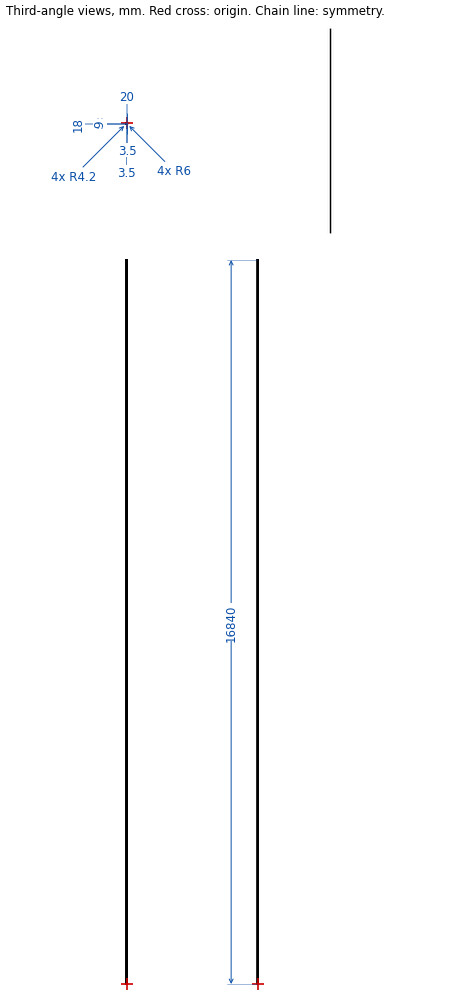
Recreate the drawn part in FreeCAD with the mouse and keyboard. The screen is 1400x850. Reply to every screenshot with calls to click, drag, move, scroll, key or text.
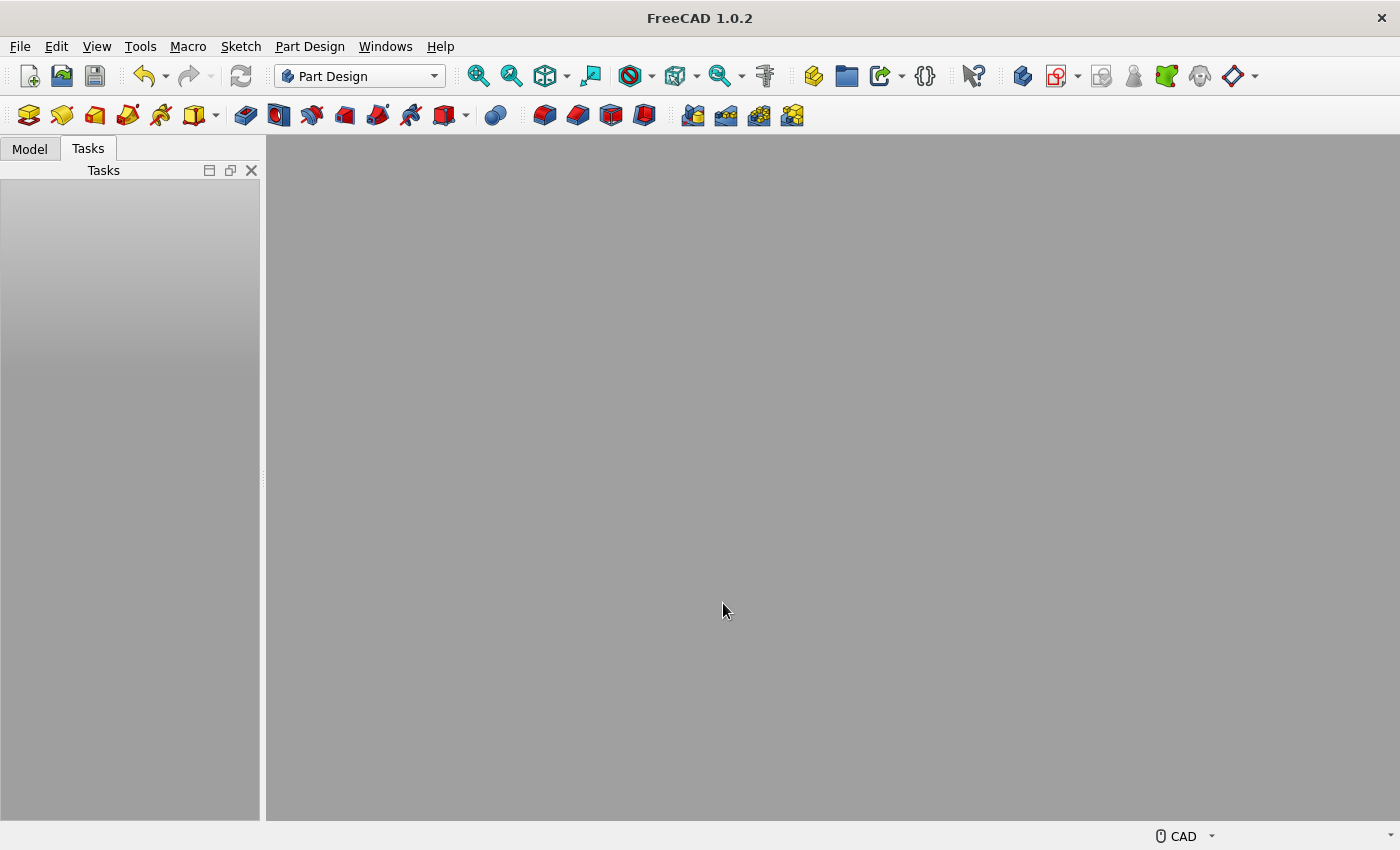
click(29, 76)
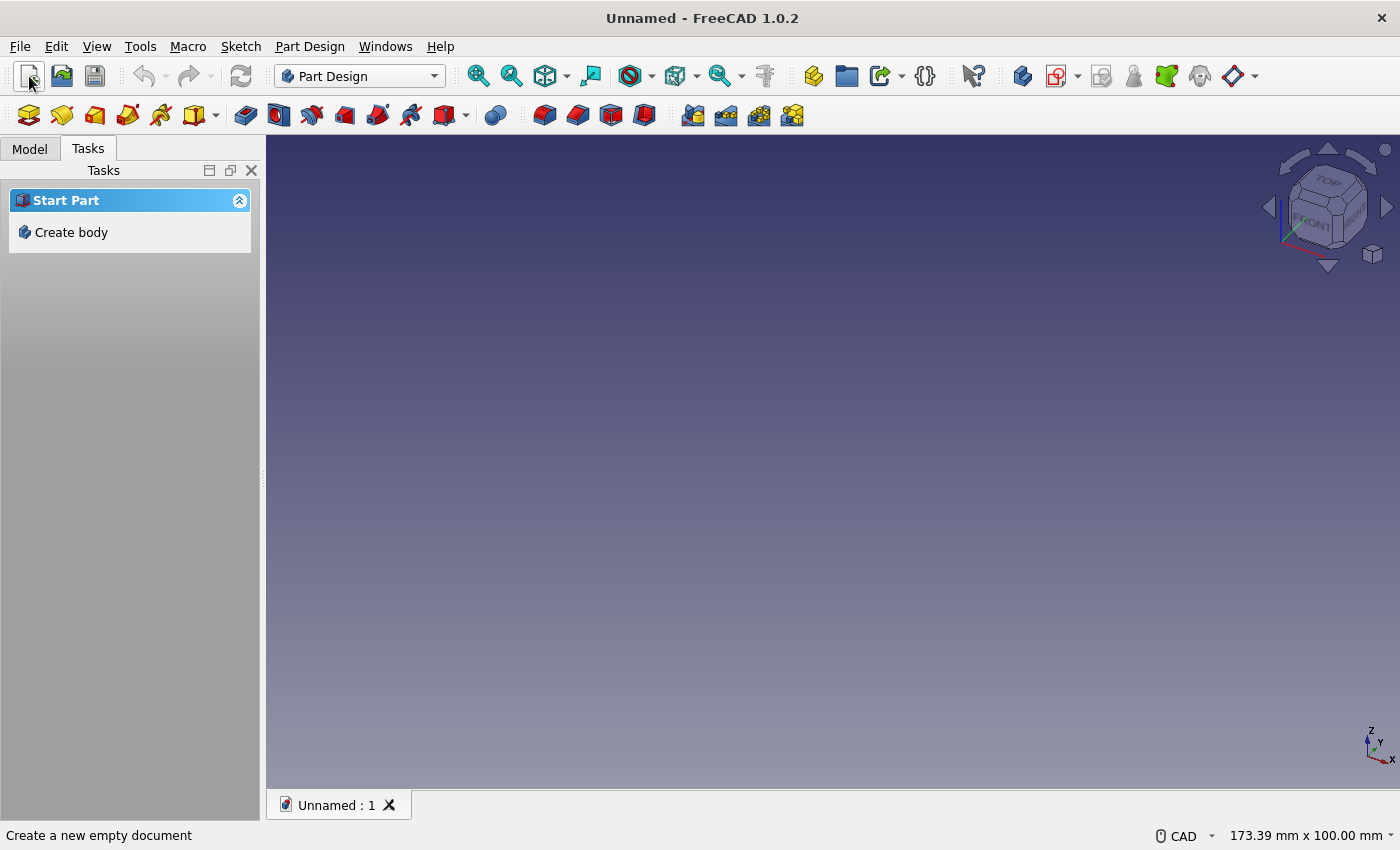
click(1056, 76)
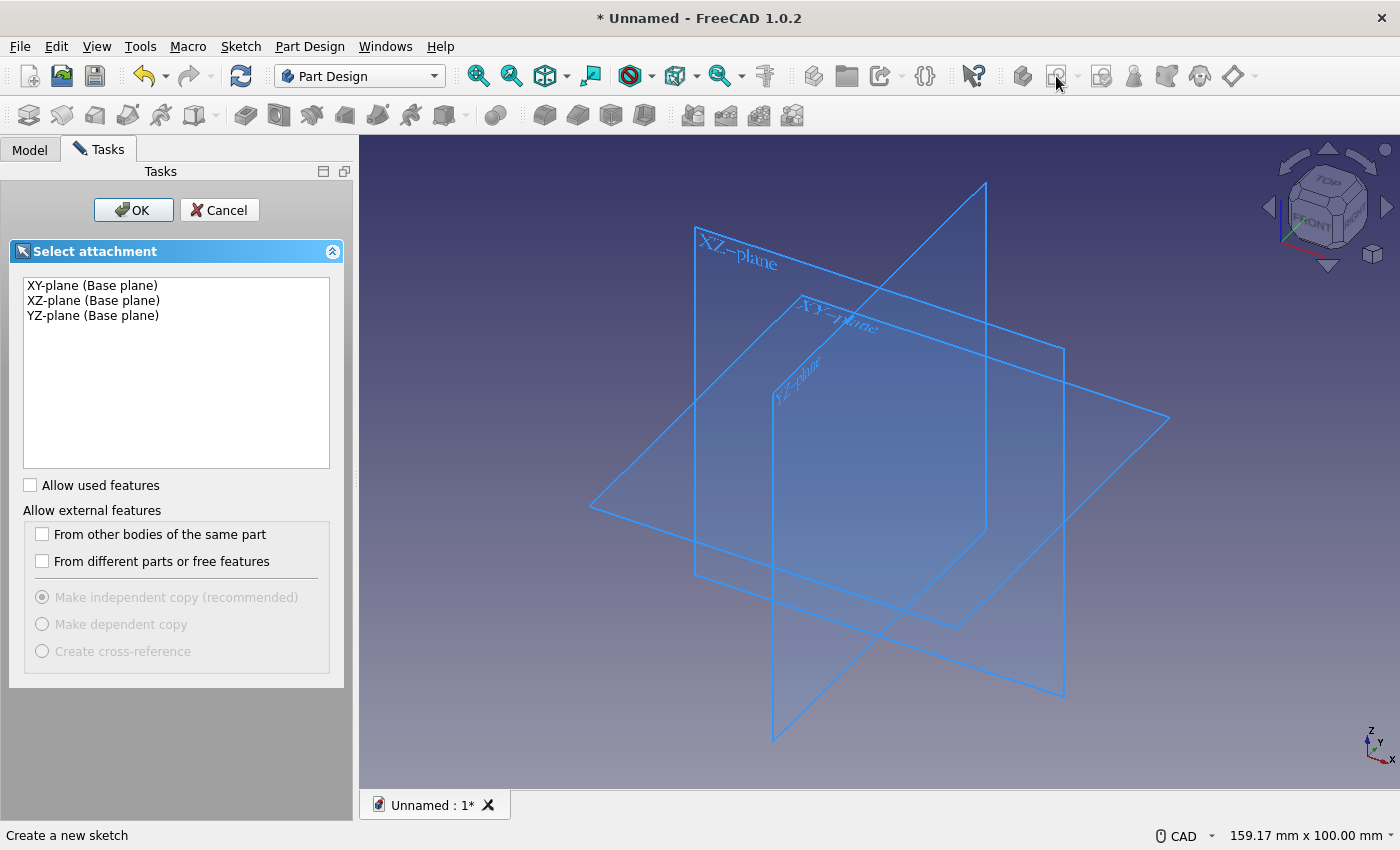
click(84, 286)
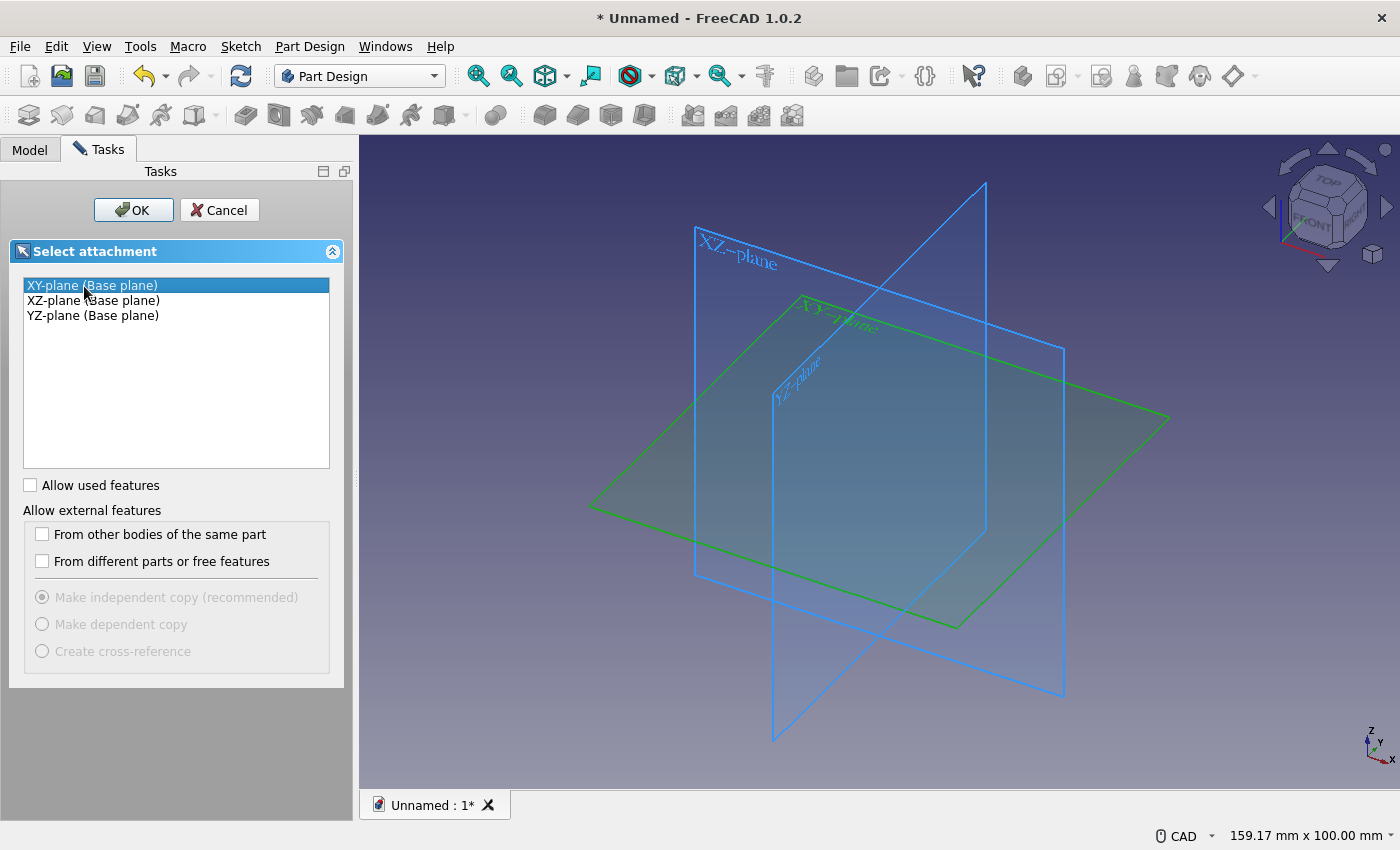
click(134, 210)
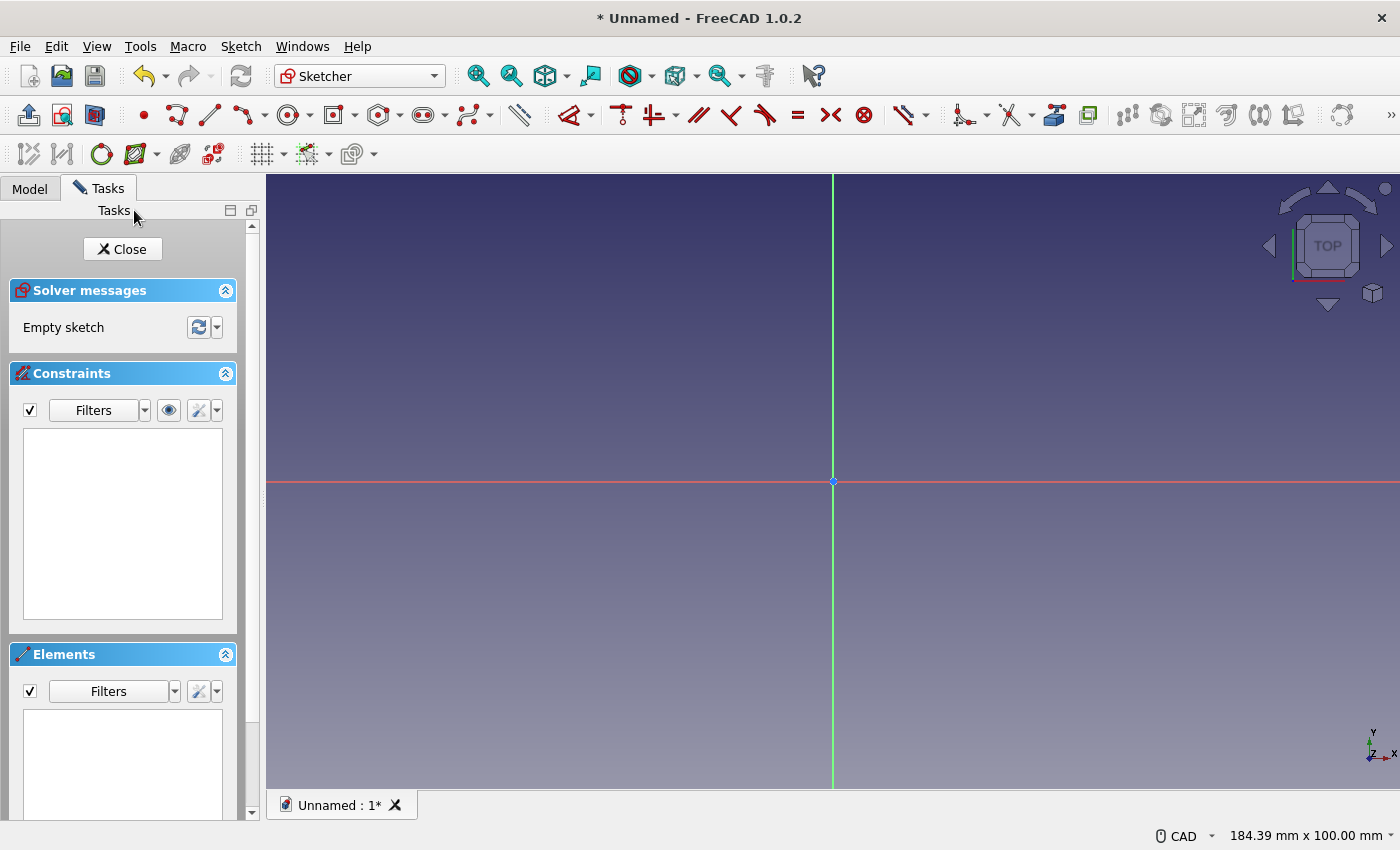
scroll(889, 482, up, 4)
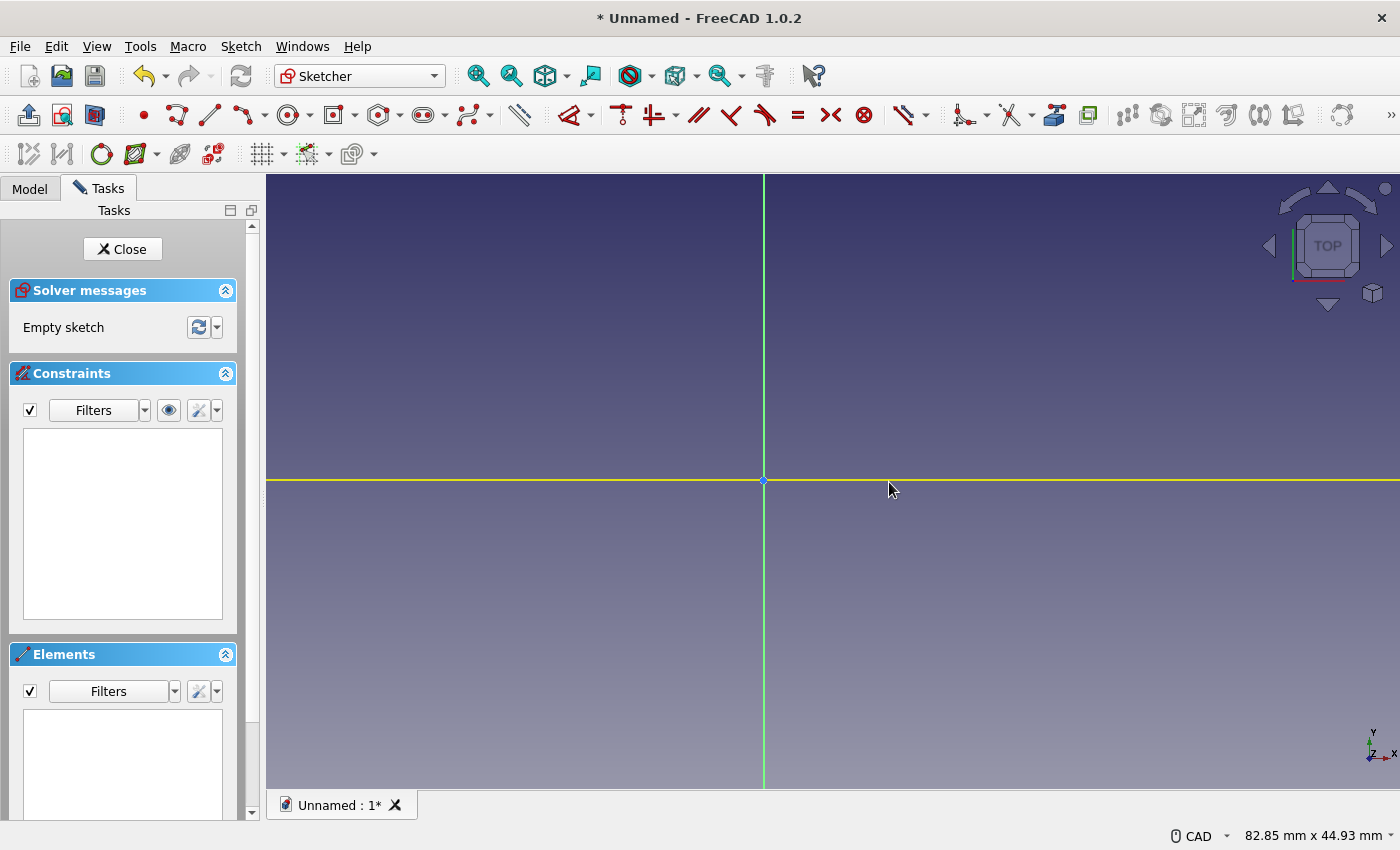
click(210, 116)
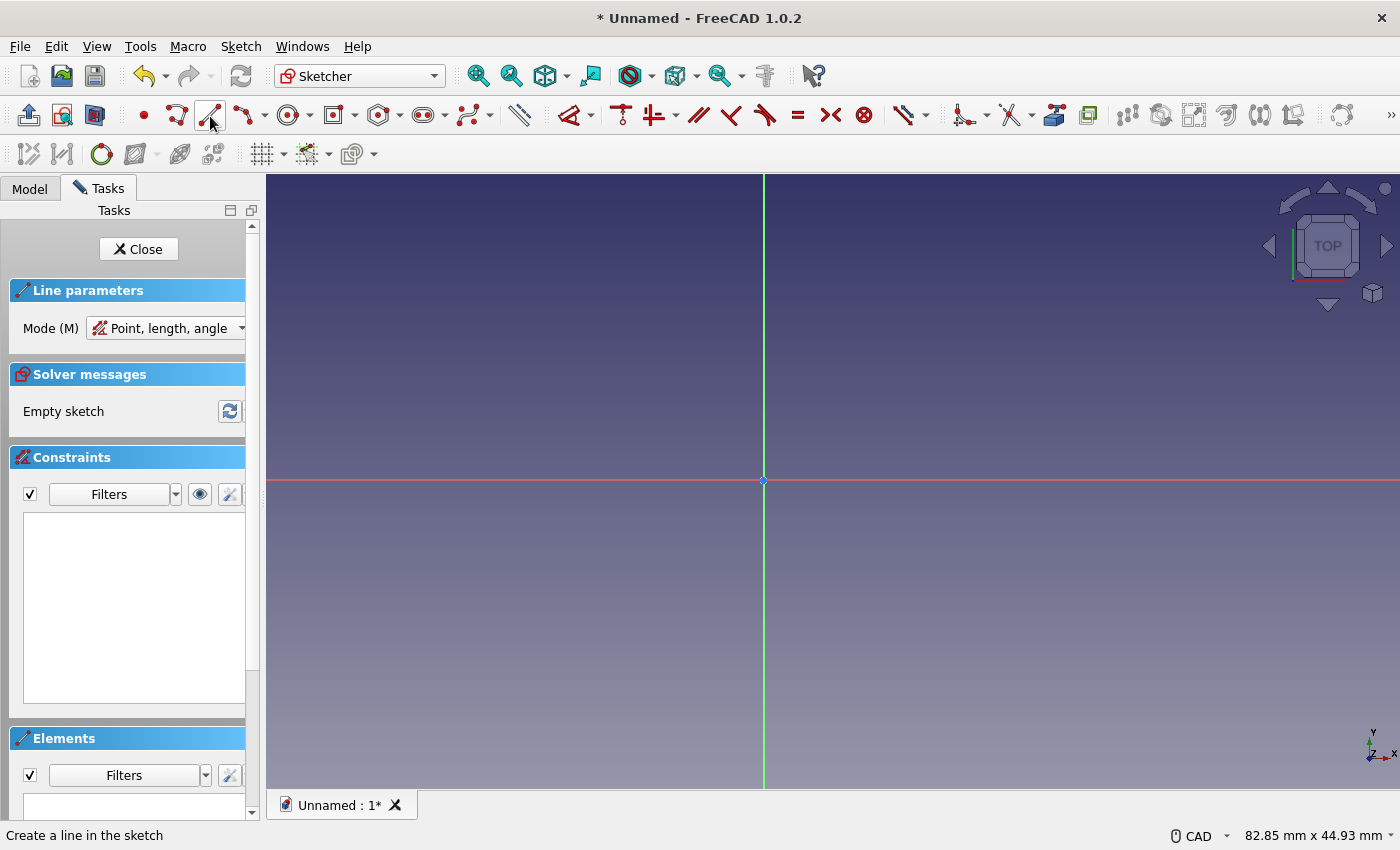
click(569, 603)
click(569, 357)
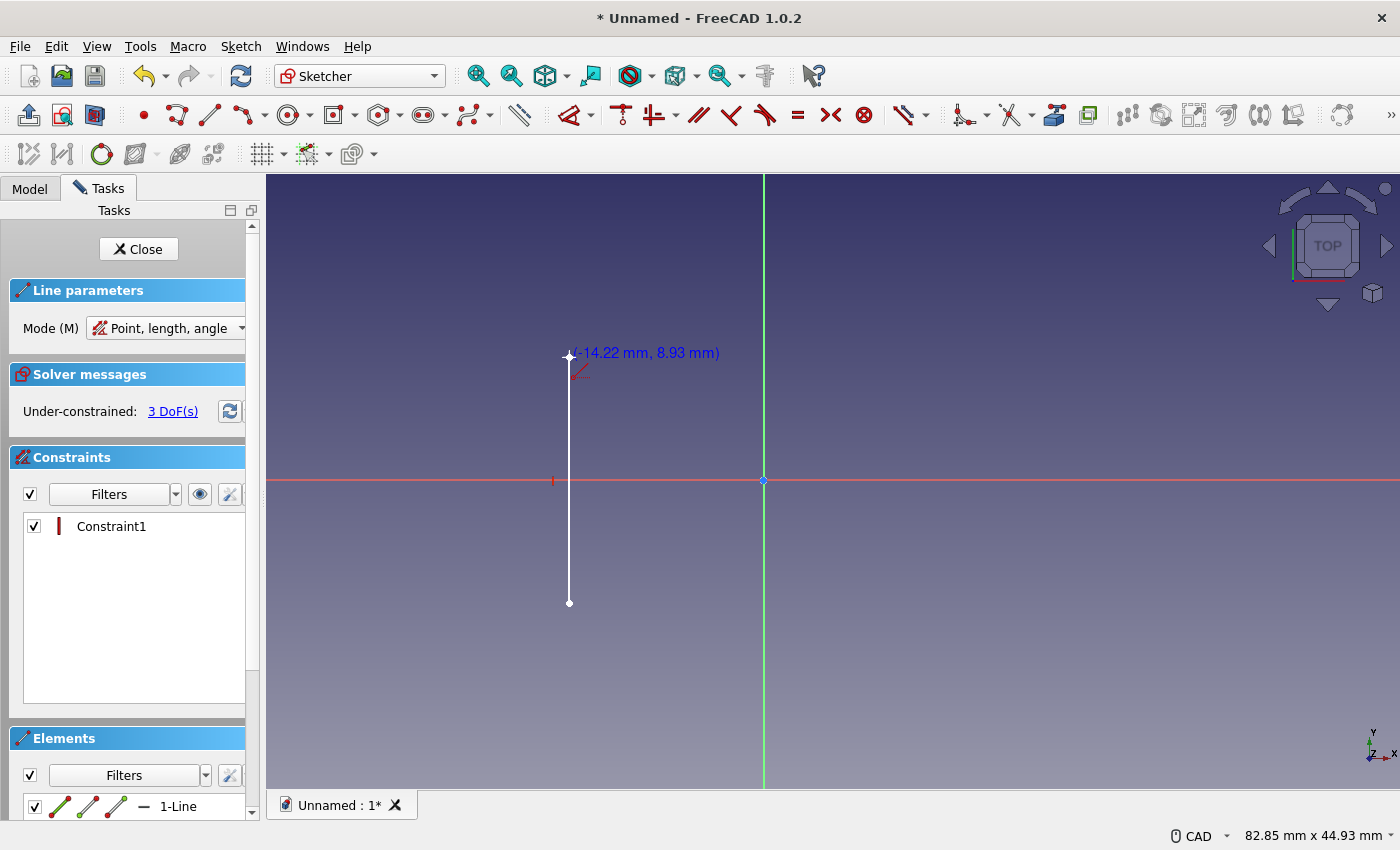
click(627, 300)
click(901, 300)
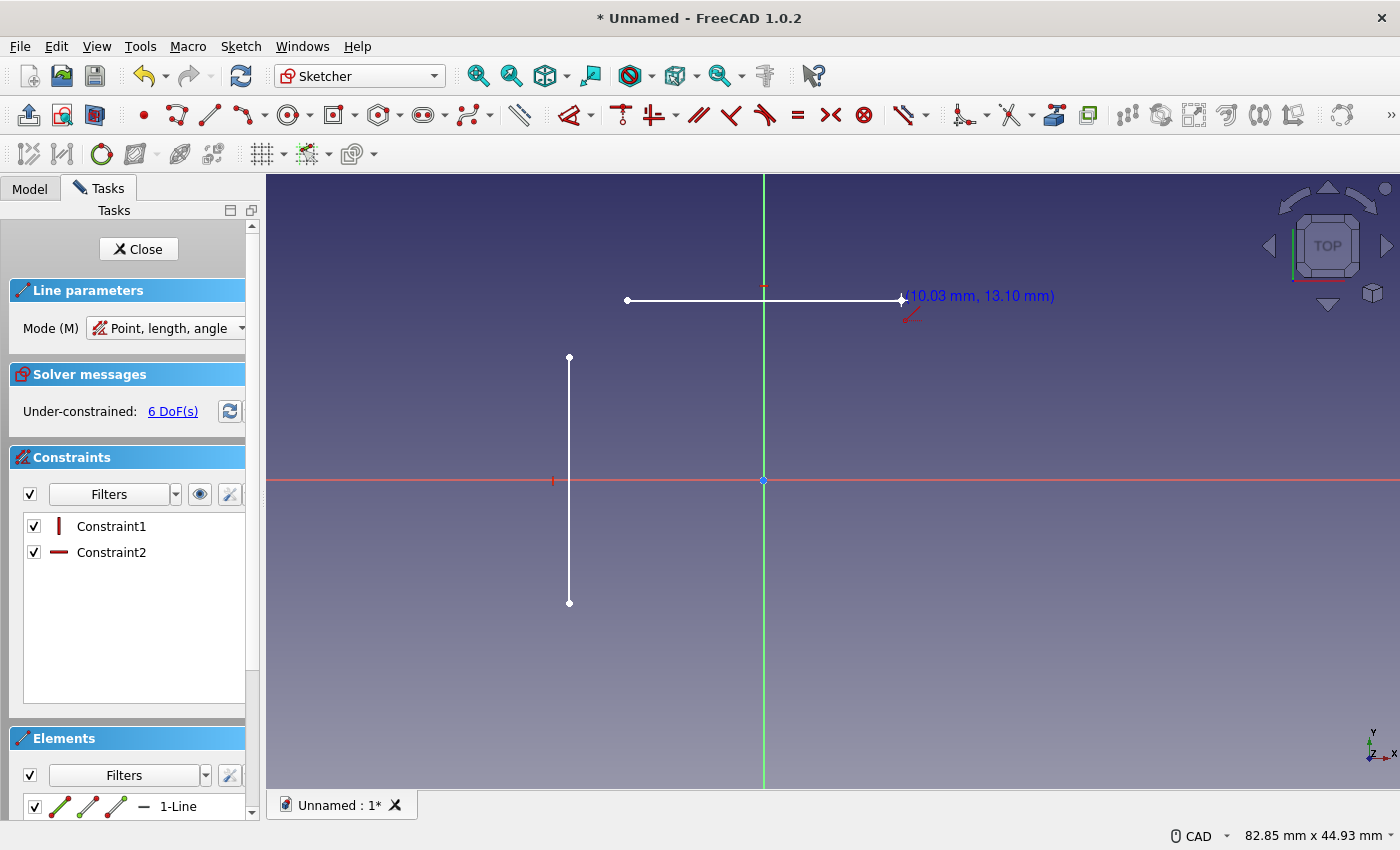
click(958, 357)
click(958, 603)